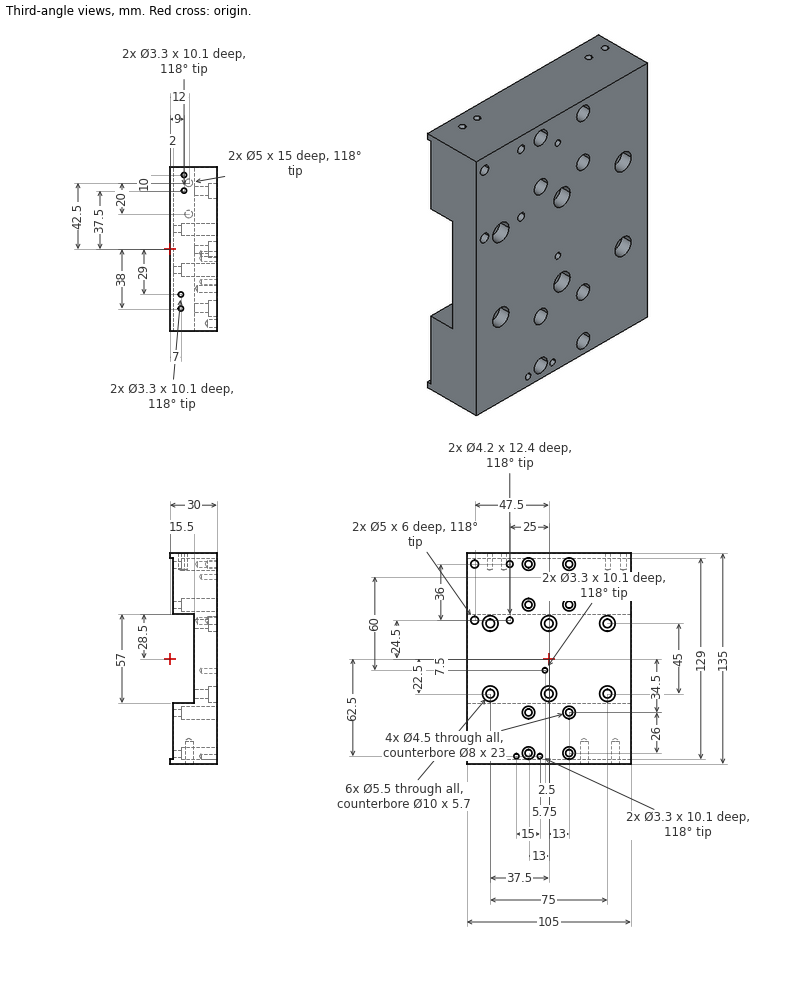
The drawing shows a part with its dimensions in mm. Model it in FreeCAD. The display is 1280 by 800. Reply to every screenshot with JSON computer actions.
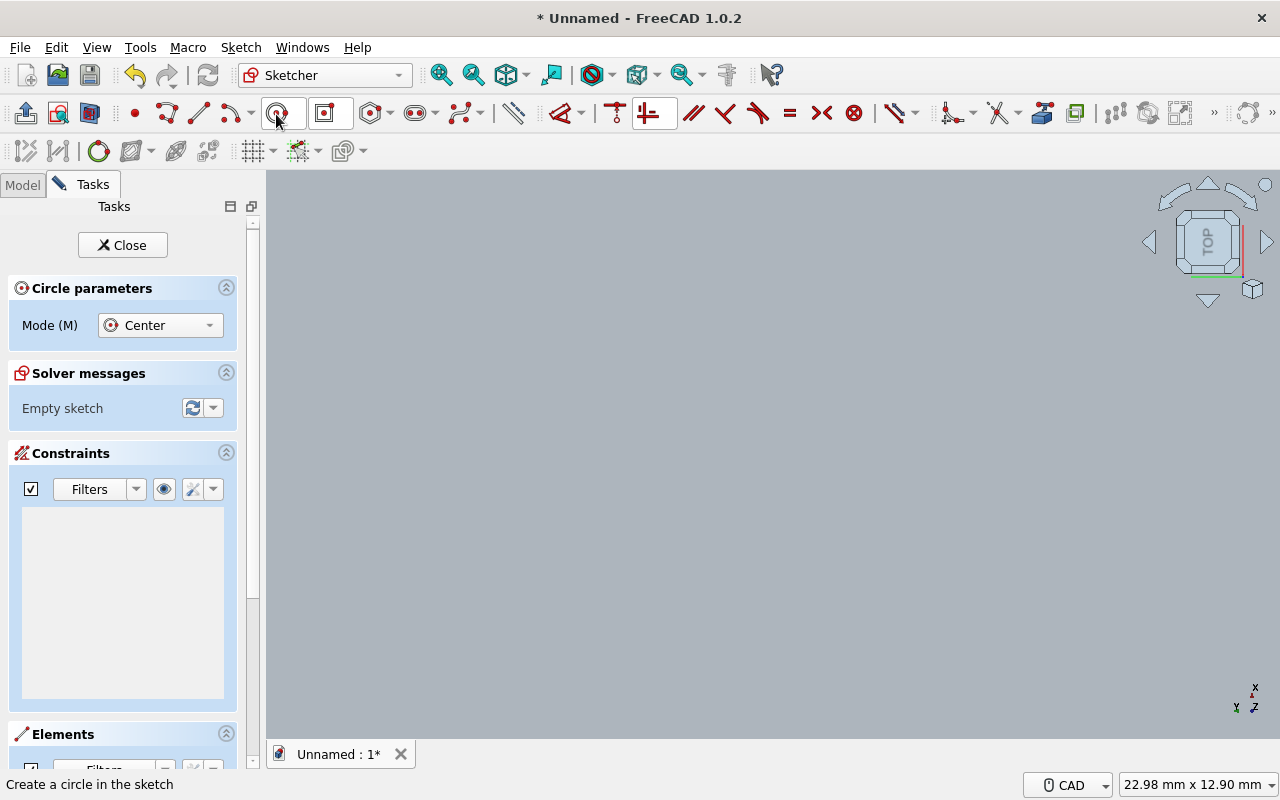
{"action": "left_click", "coordinate": [499, 445]}
{"action": "left_click", "coordinate": [551, 394]}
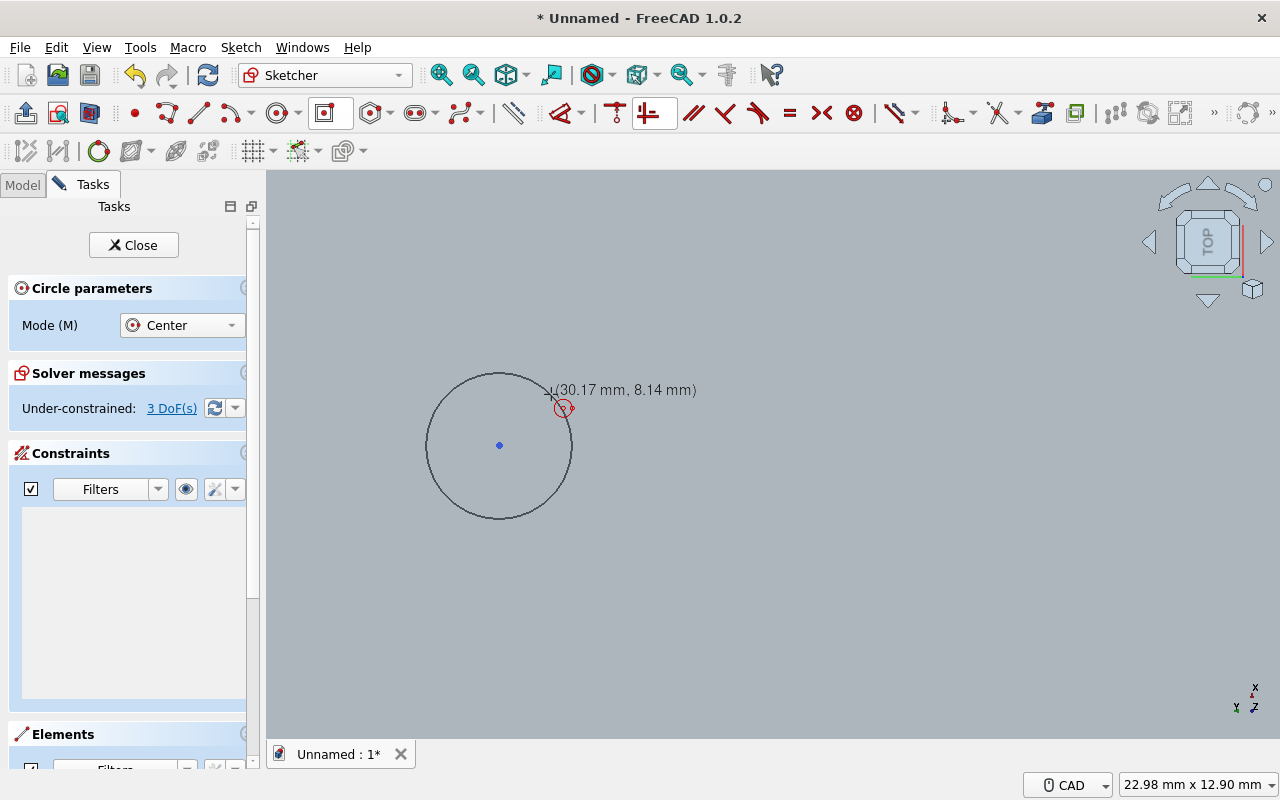
{"action": "left_click", "coordinate": [896, 445]}
{"action": "left_click", "coordinate": [948, 394]}
{"action": "key", "text": "Escape"}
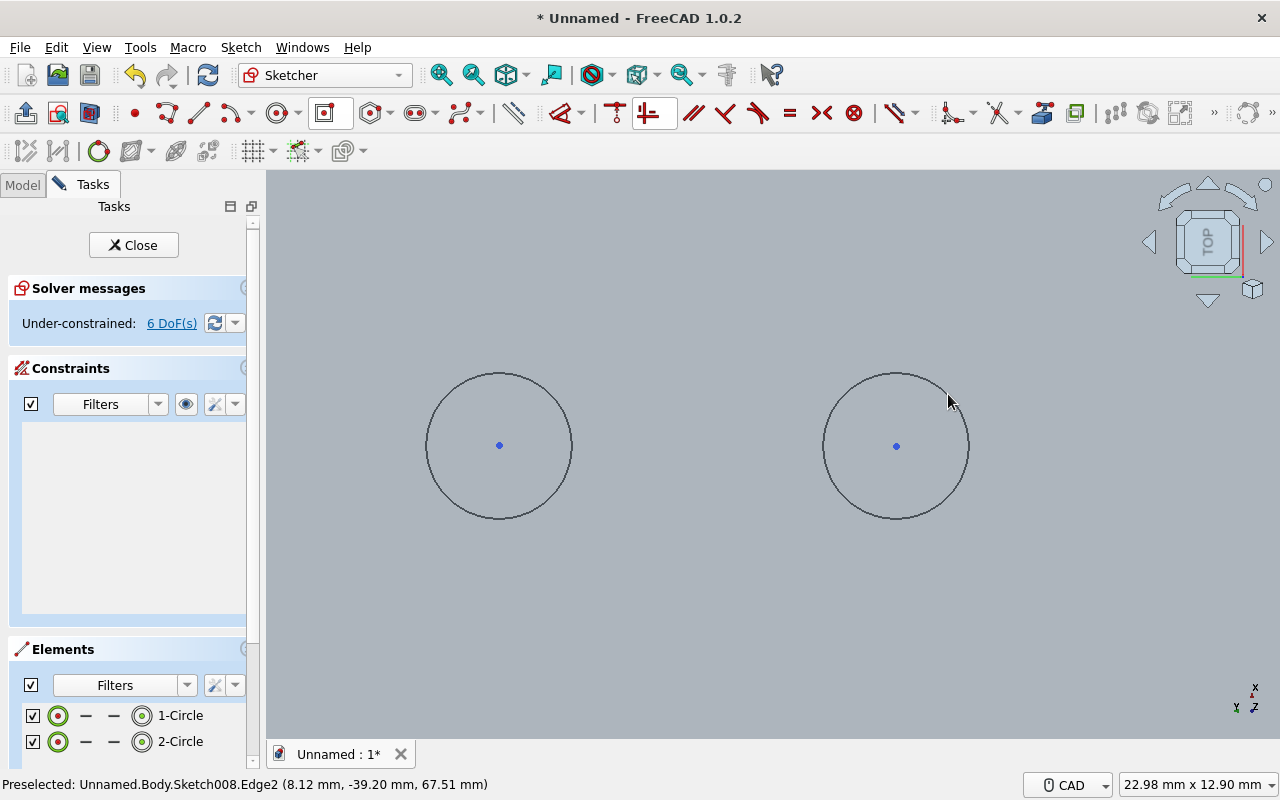
{"action": "left_click", "coordinate": [550, 394]}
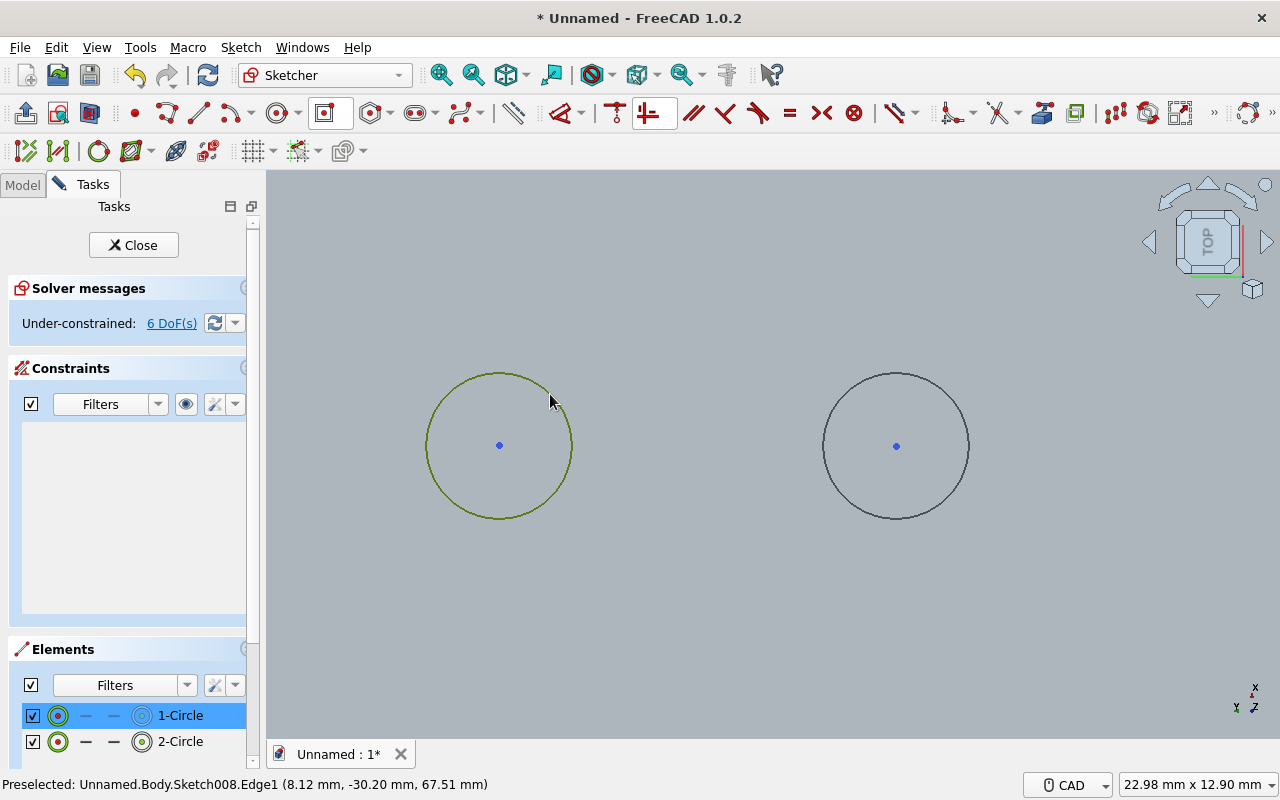
{"action": "left_click", "coordinate": [947, 394]}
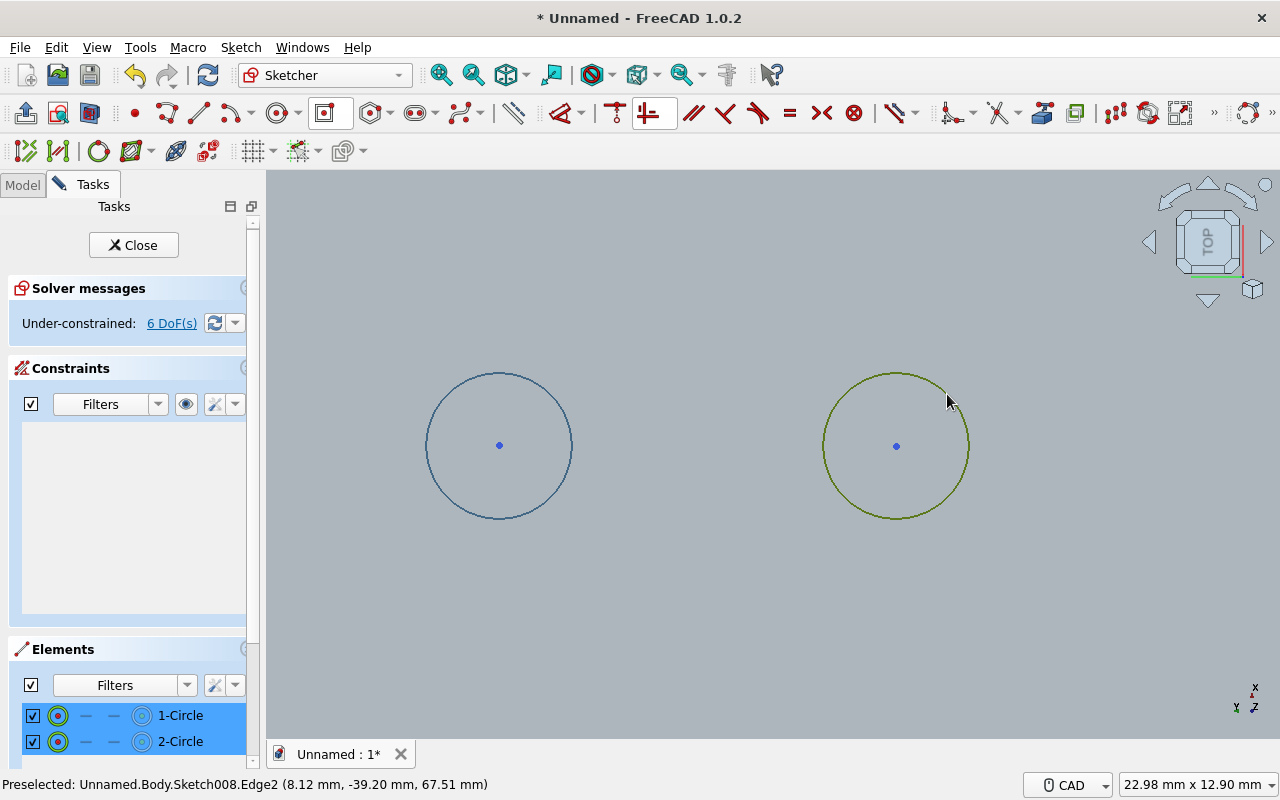
{"action": "left_click", "coordinate": [790, 114]}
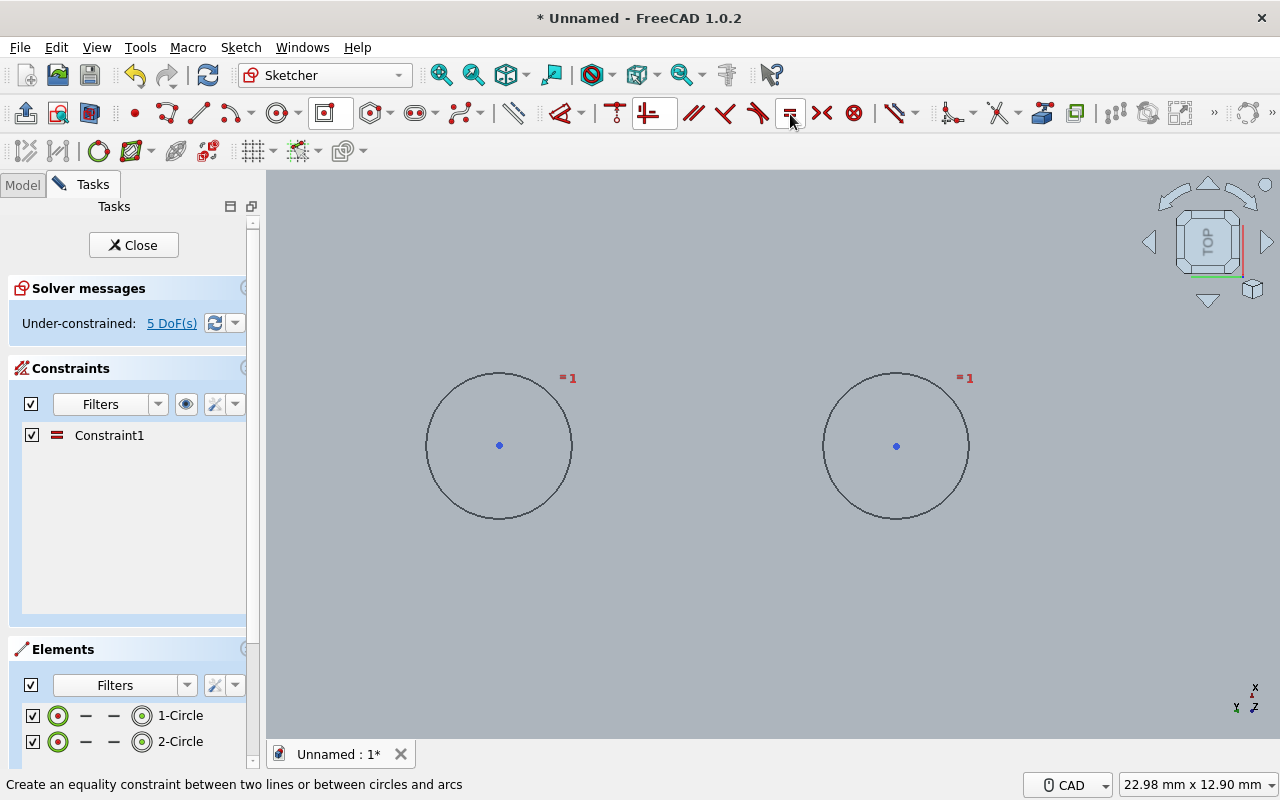
{"action": "left_click", "coordinate": [499, 446]}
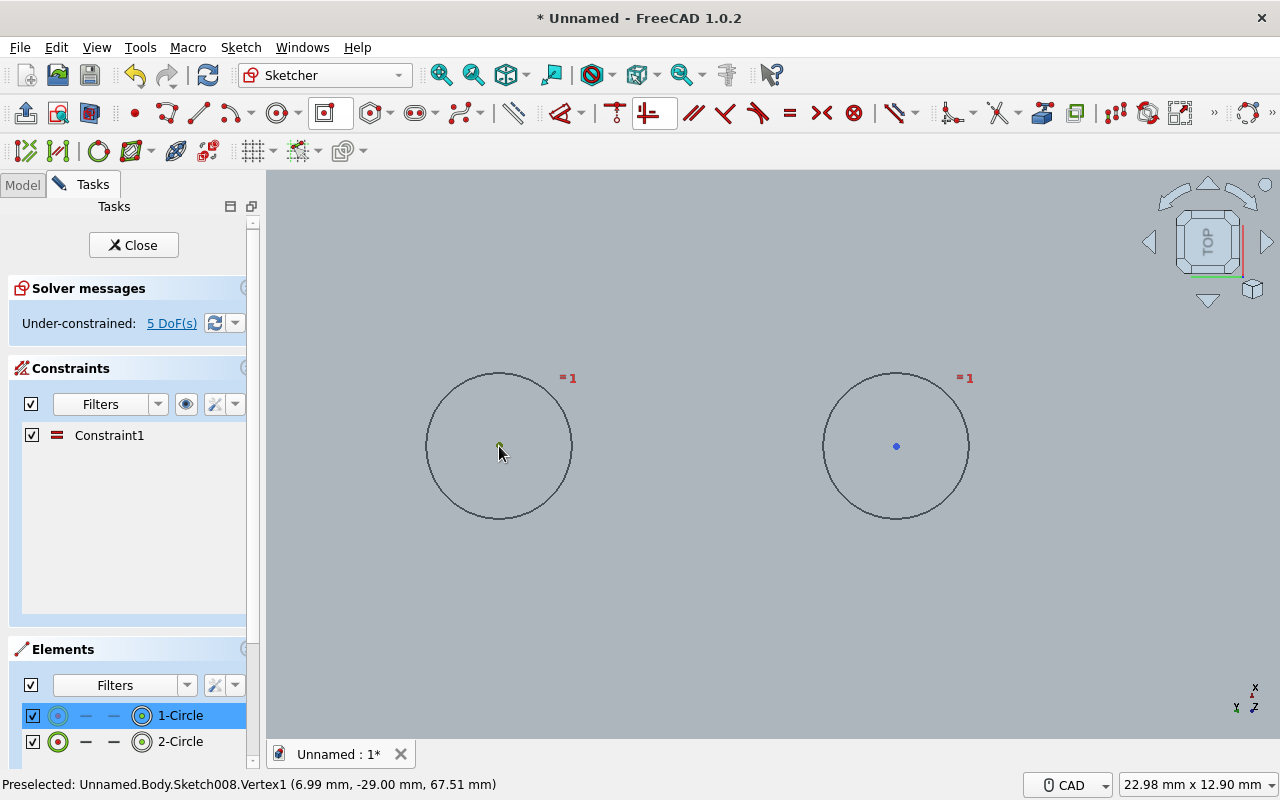
{"action": "left_click", "coordinate": [896, 446]}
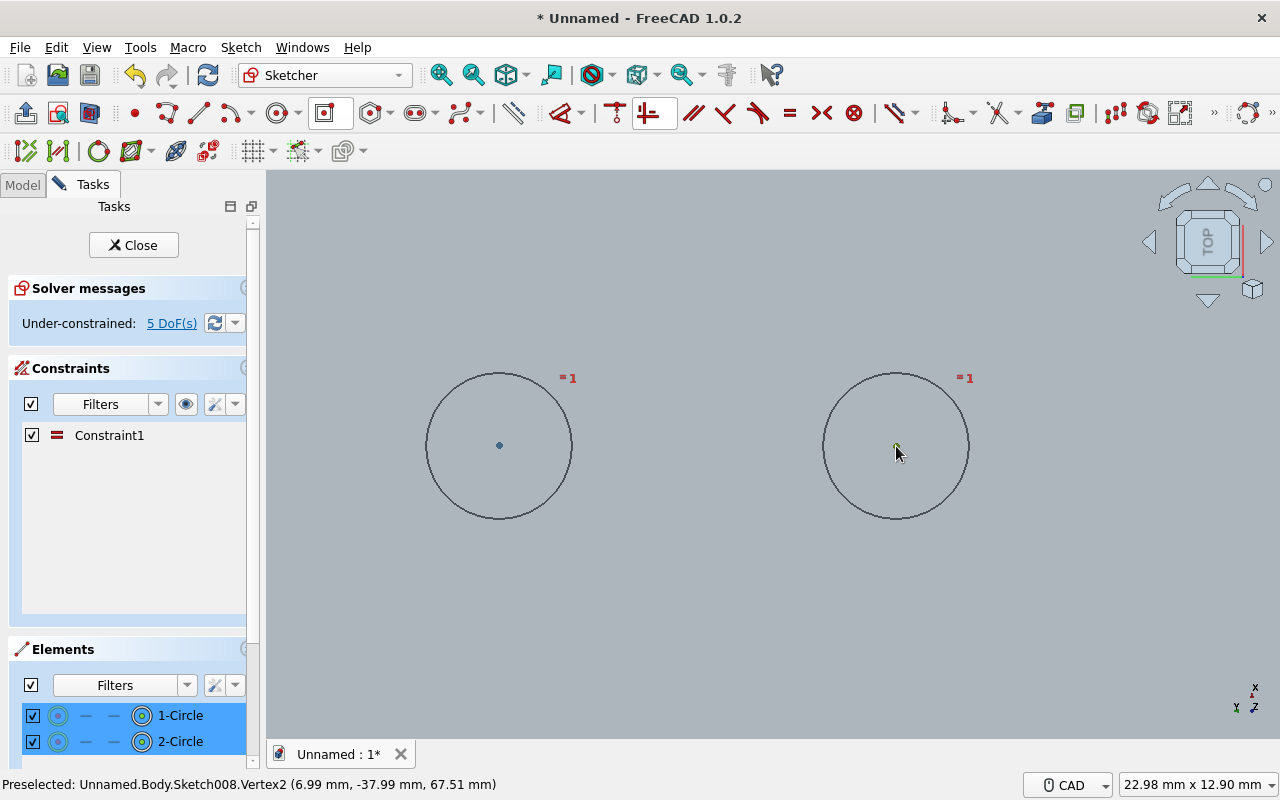
{"action": "key", "text": "h"}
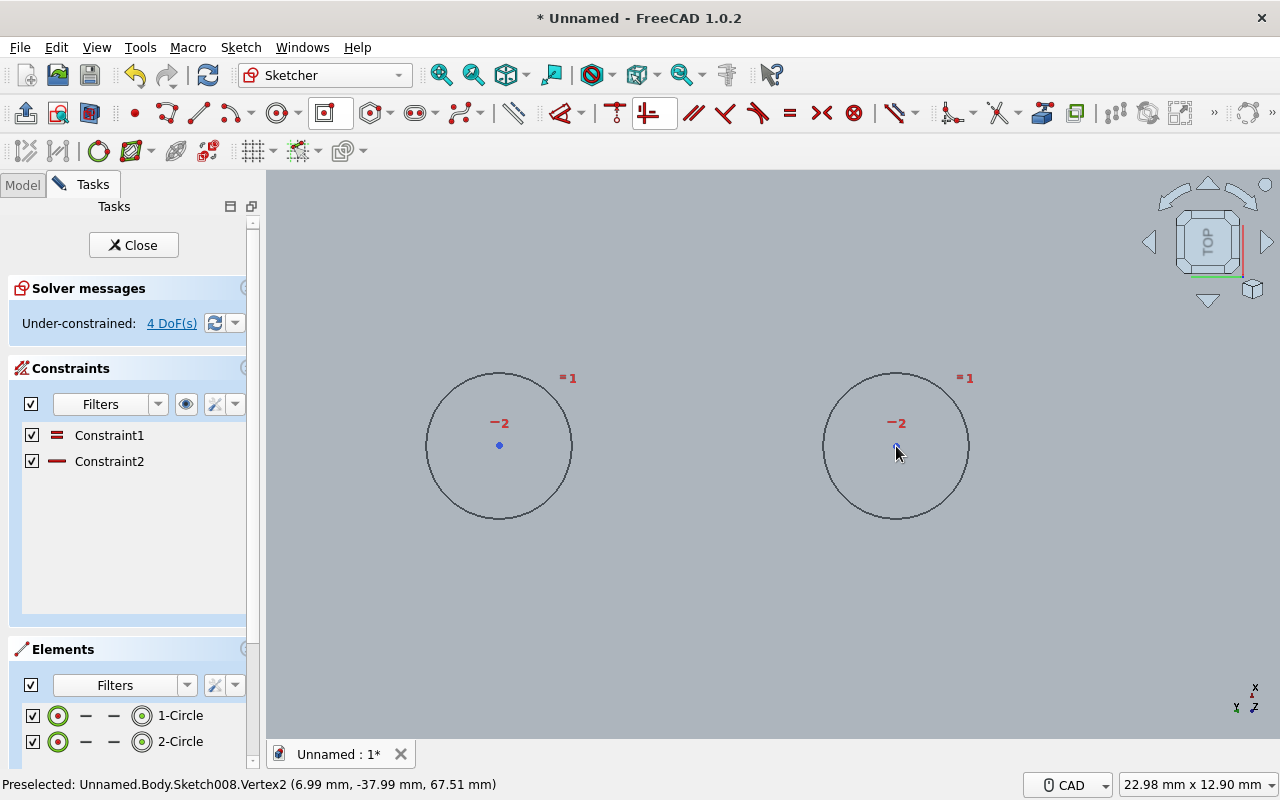
{"action": "left_click", "coordinate": [560, 114]}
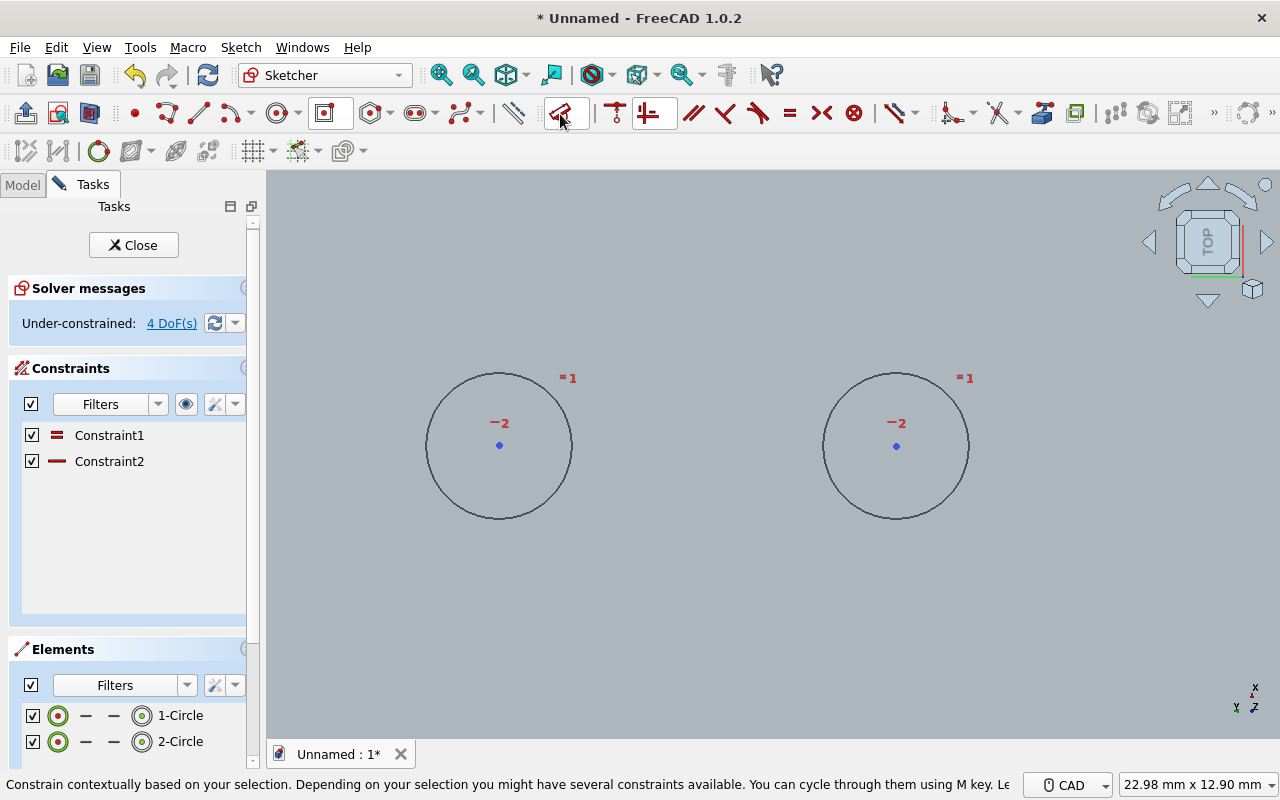
{"action": "left_click", "coordinate": [550, 394]}
{"action": "left_click", "coordinate": [572, 371]}